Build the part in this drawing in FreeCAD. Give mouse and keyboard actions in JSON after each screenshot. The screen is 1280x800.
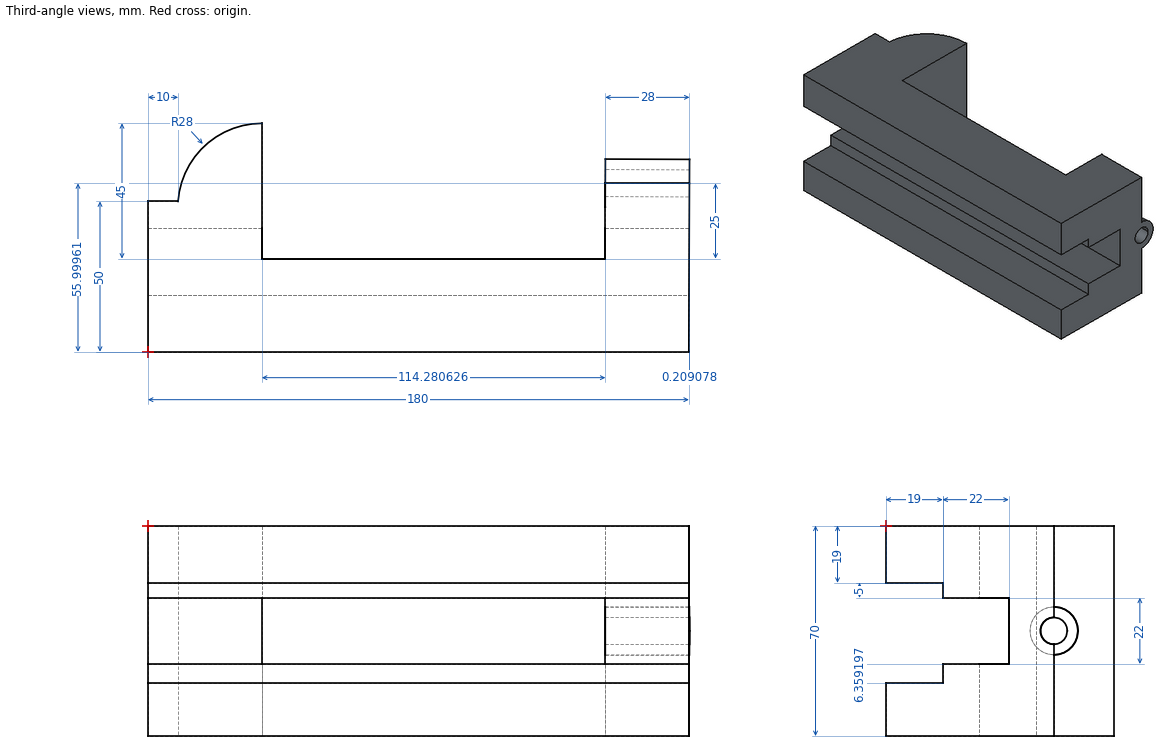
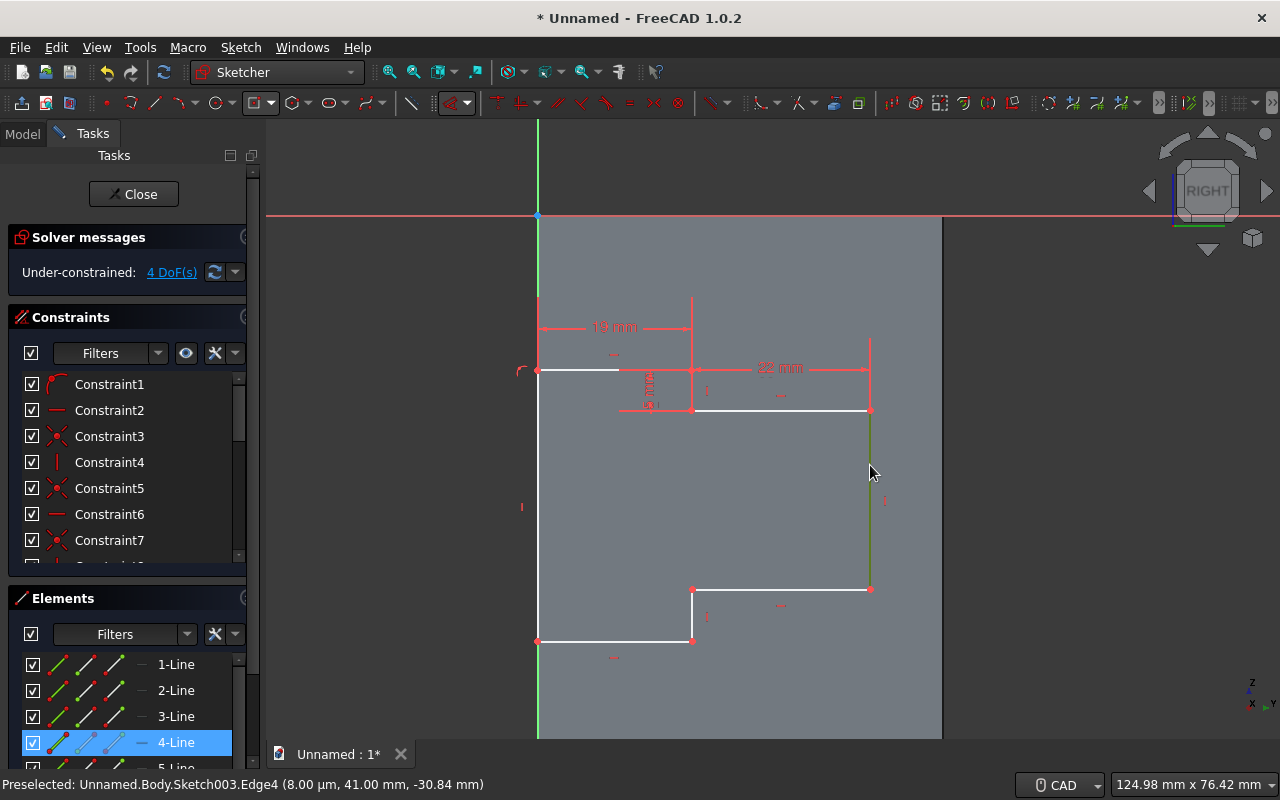
{"action": "key", "text": "i"}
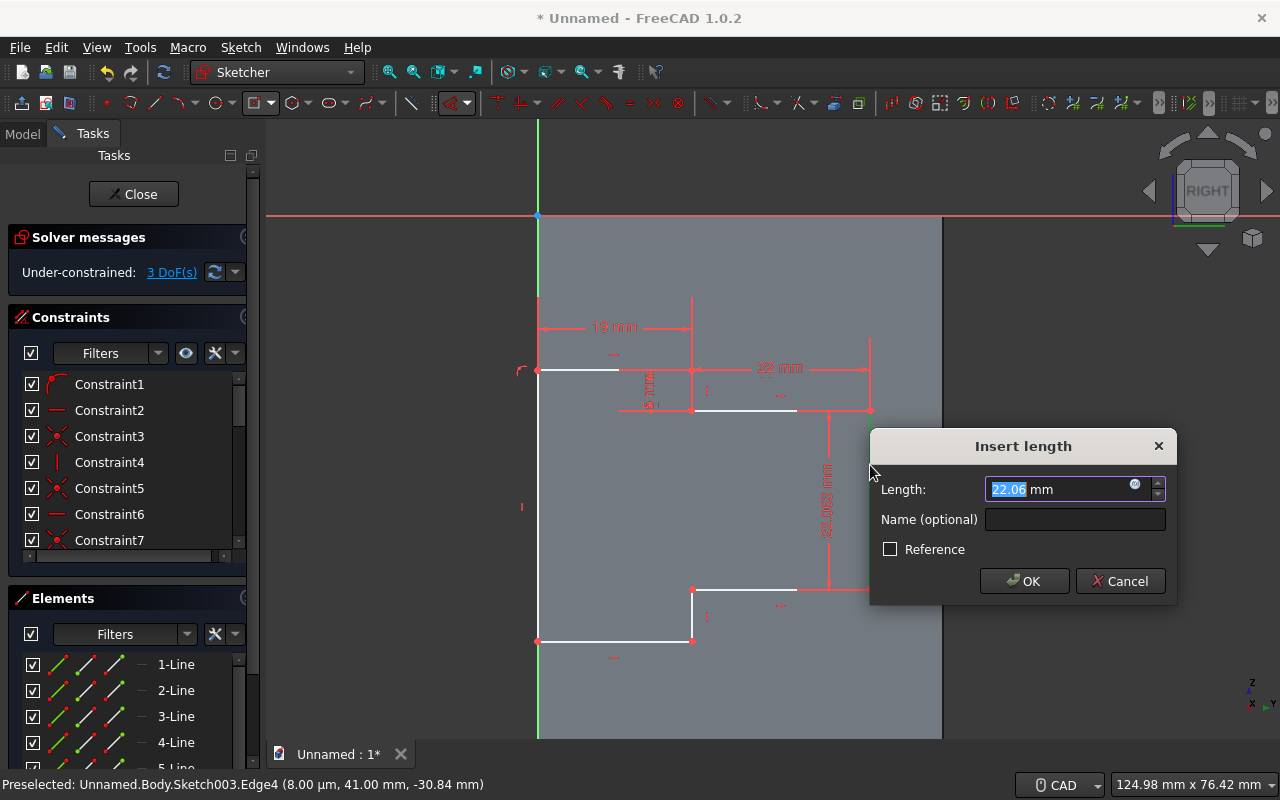
{"action": "type", "text": "22"}
{"action": "key", "text": "Return"}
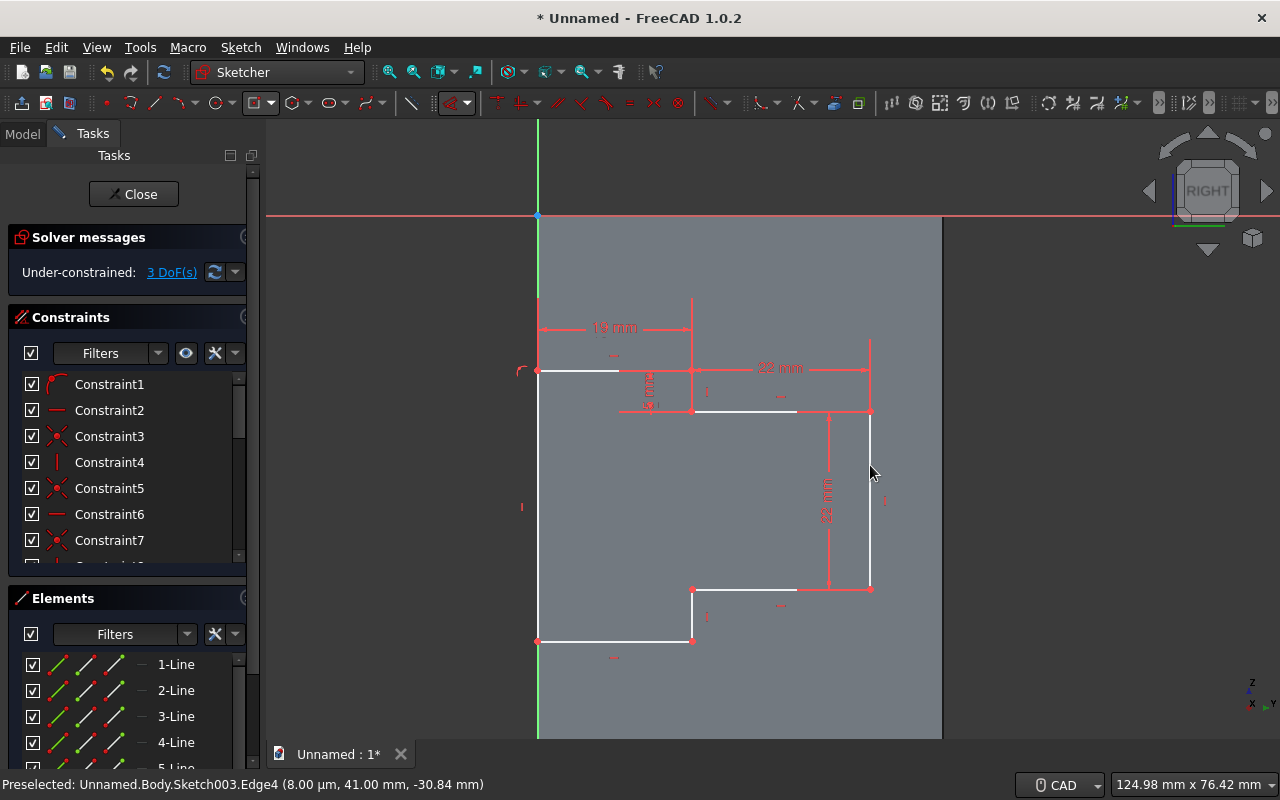
{"action": "left_click", "coordinate": [817, 590]}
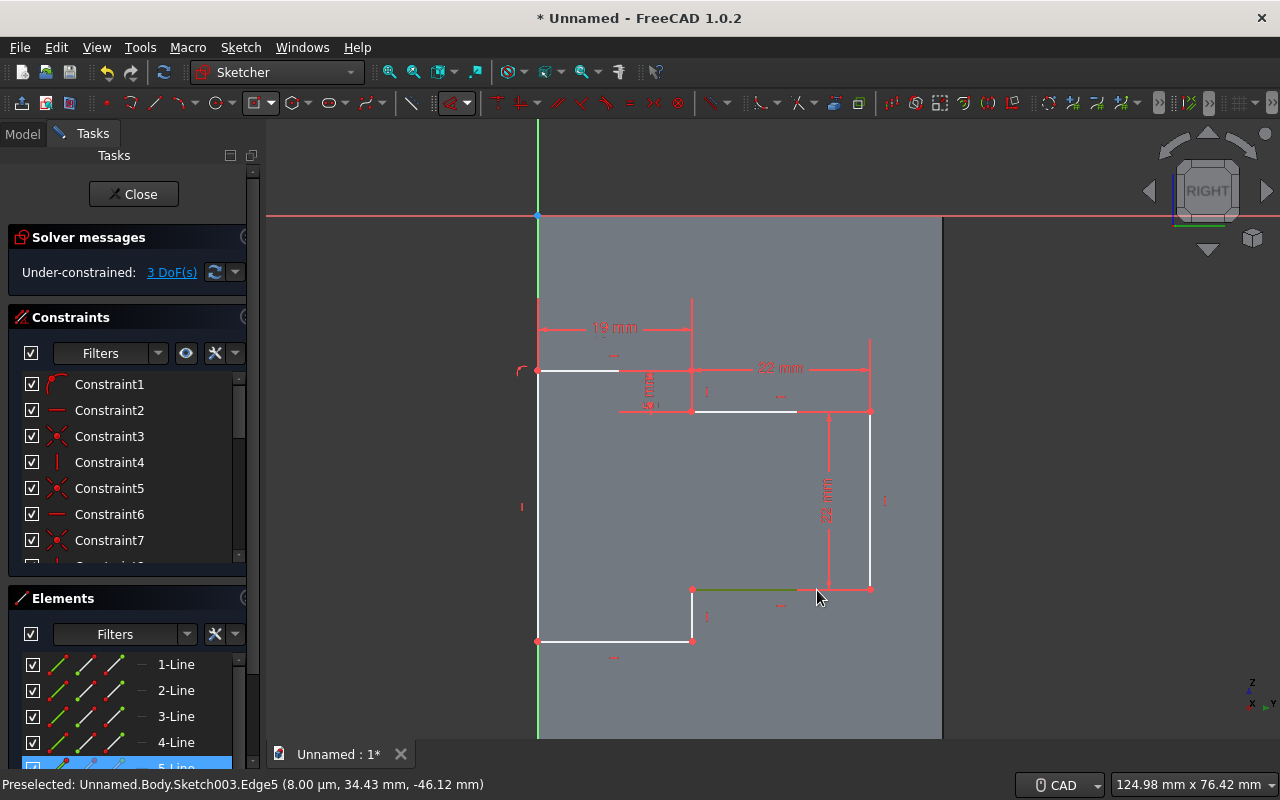
{"action": "left_click", "coordinate": [470, 104]}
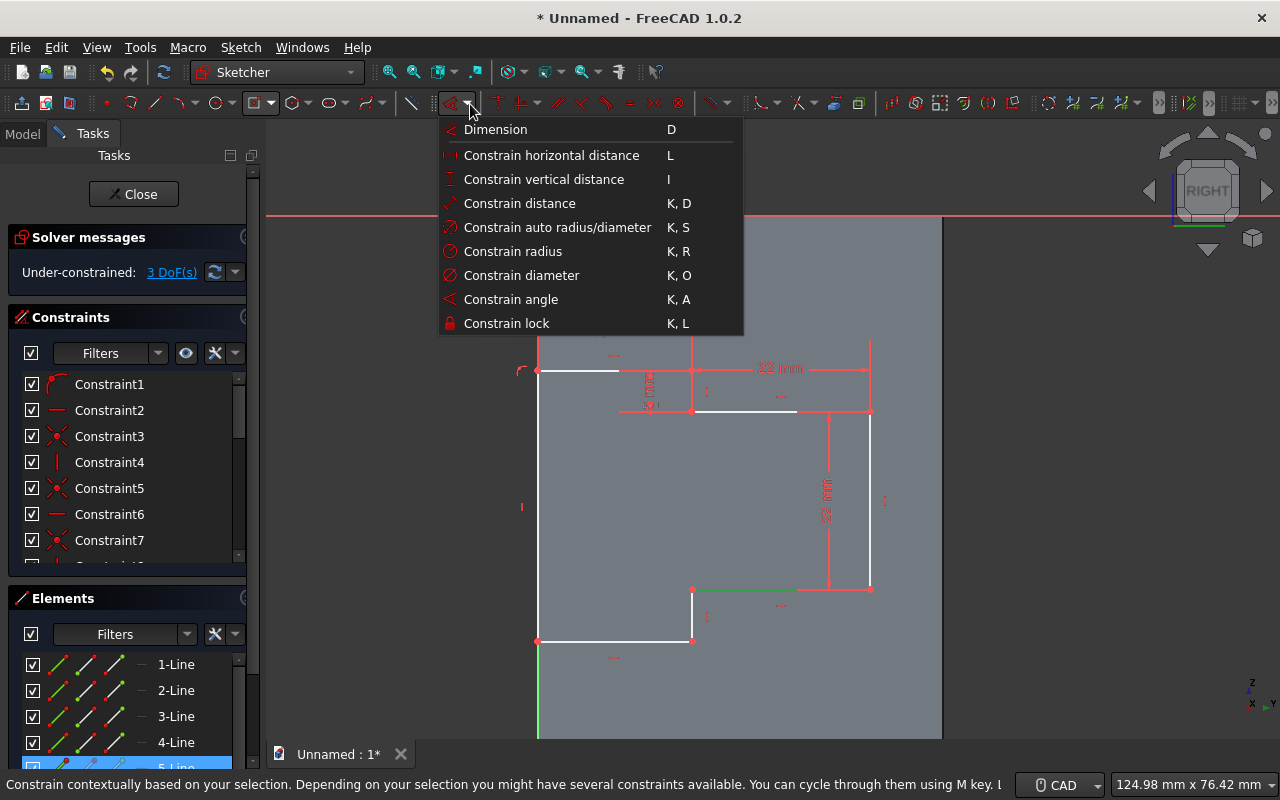
{"action": "left_click", "coordinate": [591, 155]}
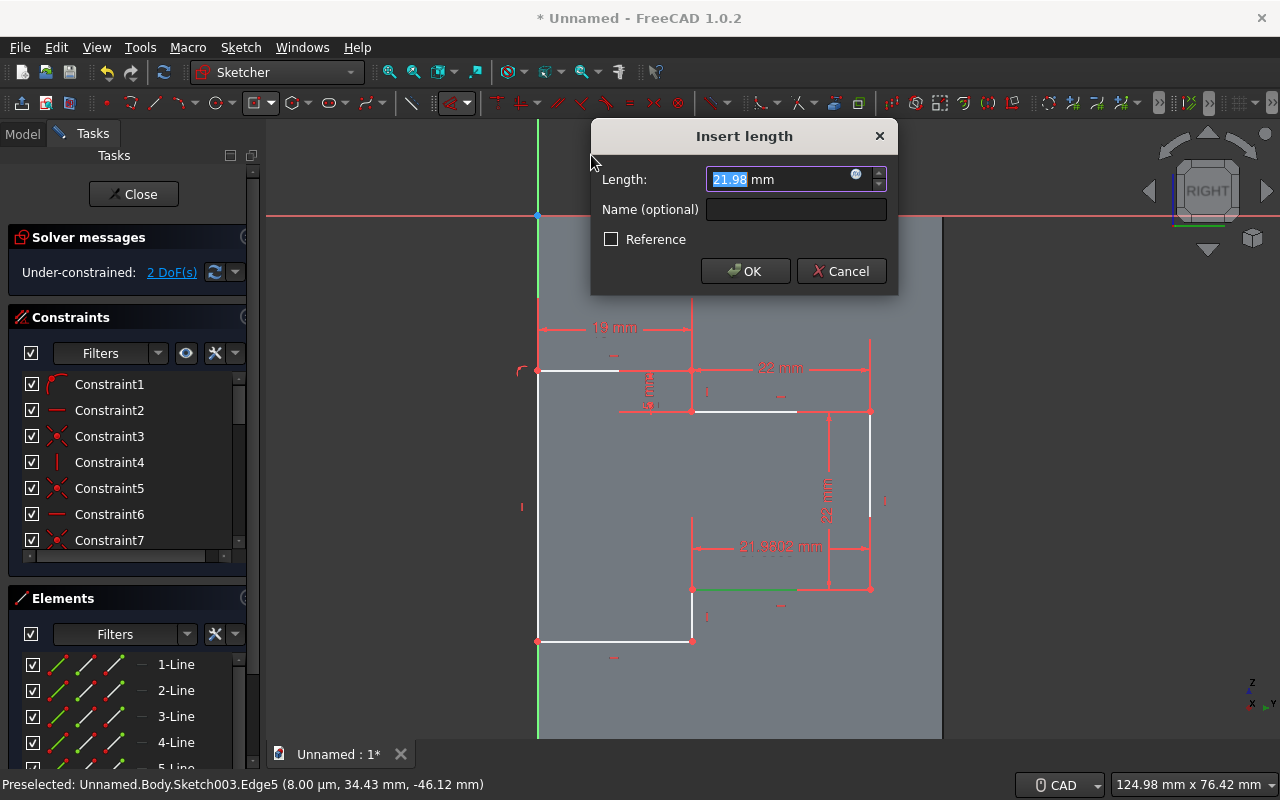
{"action": "type", "text": "22"}
{"action": "key", "text": "Return"}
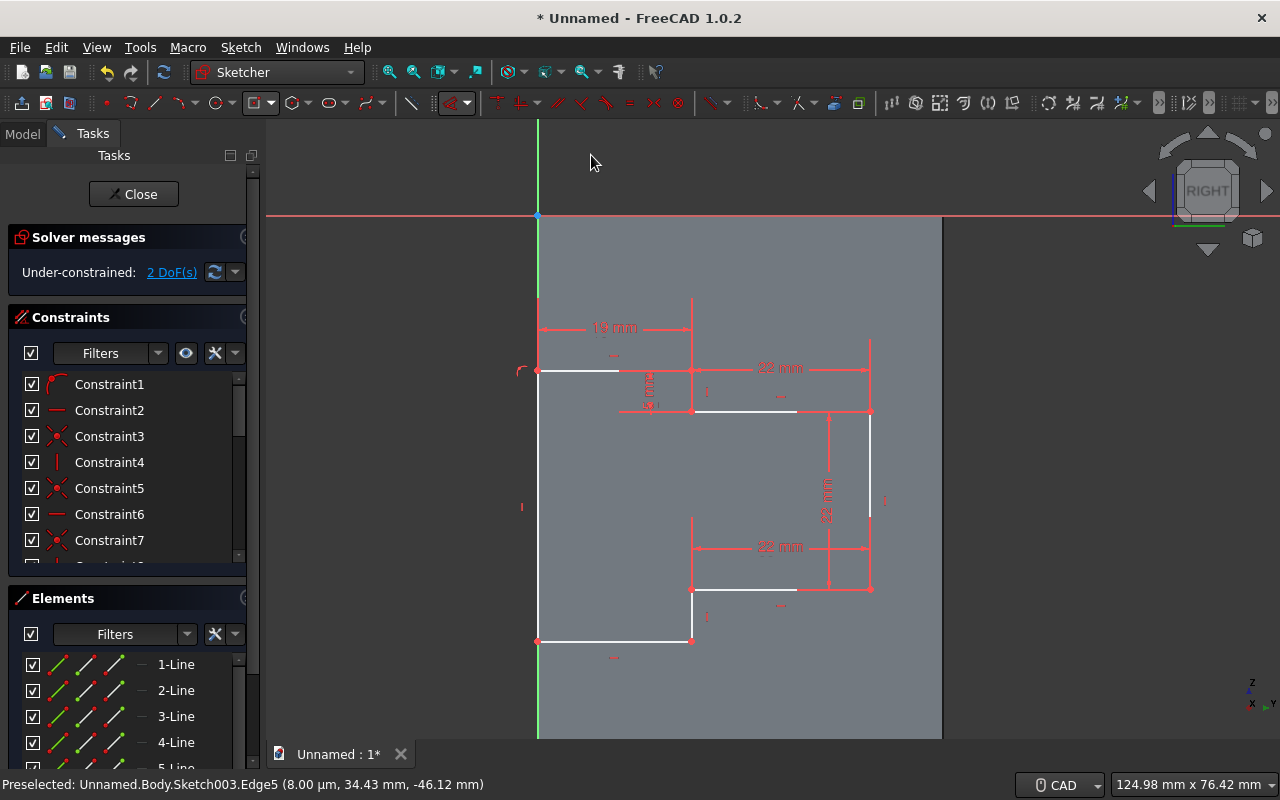
{"action": "left_click", "coordinate": [538, 371]}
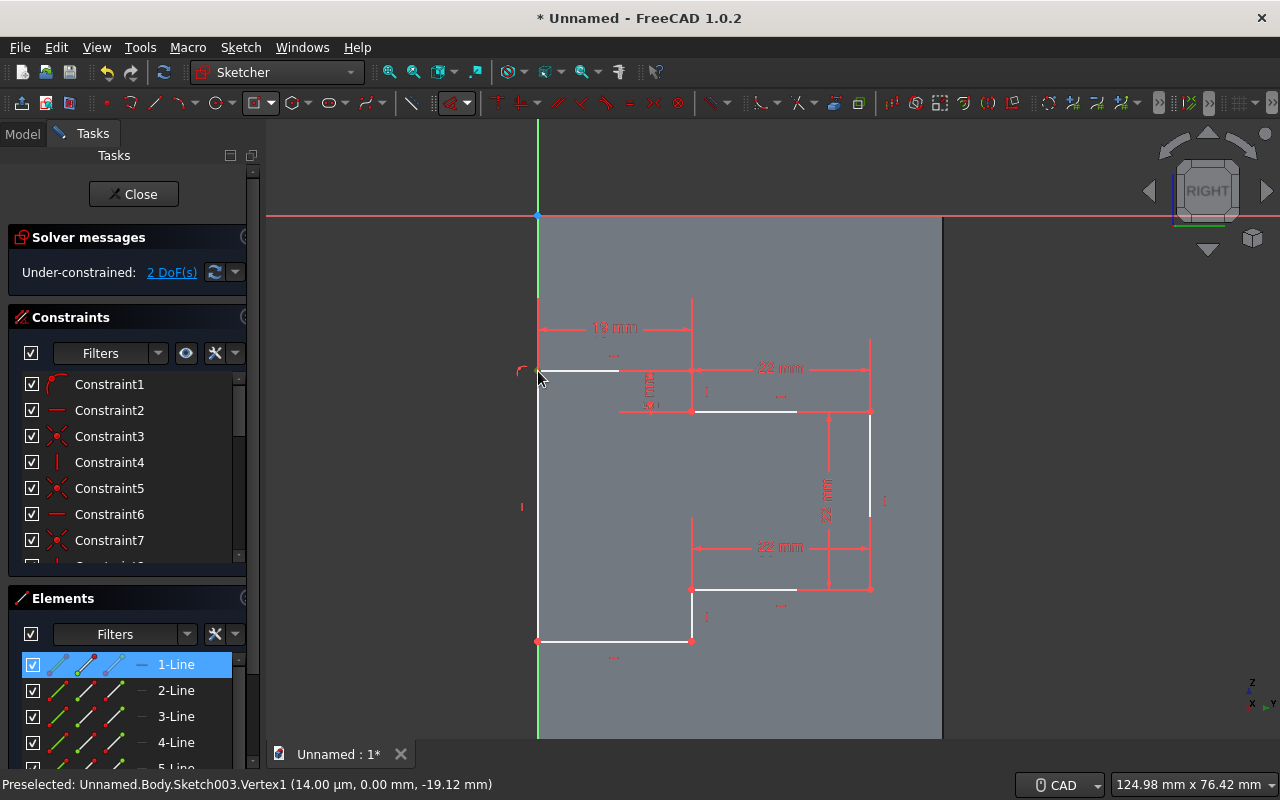
{"action": "left_click", "coordinate": [470, 104]}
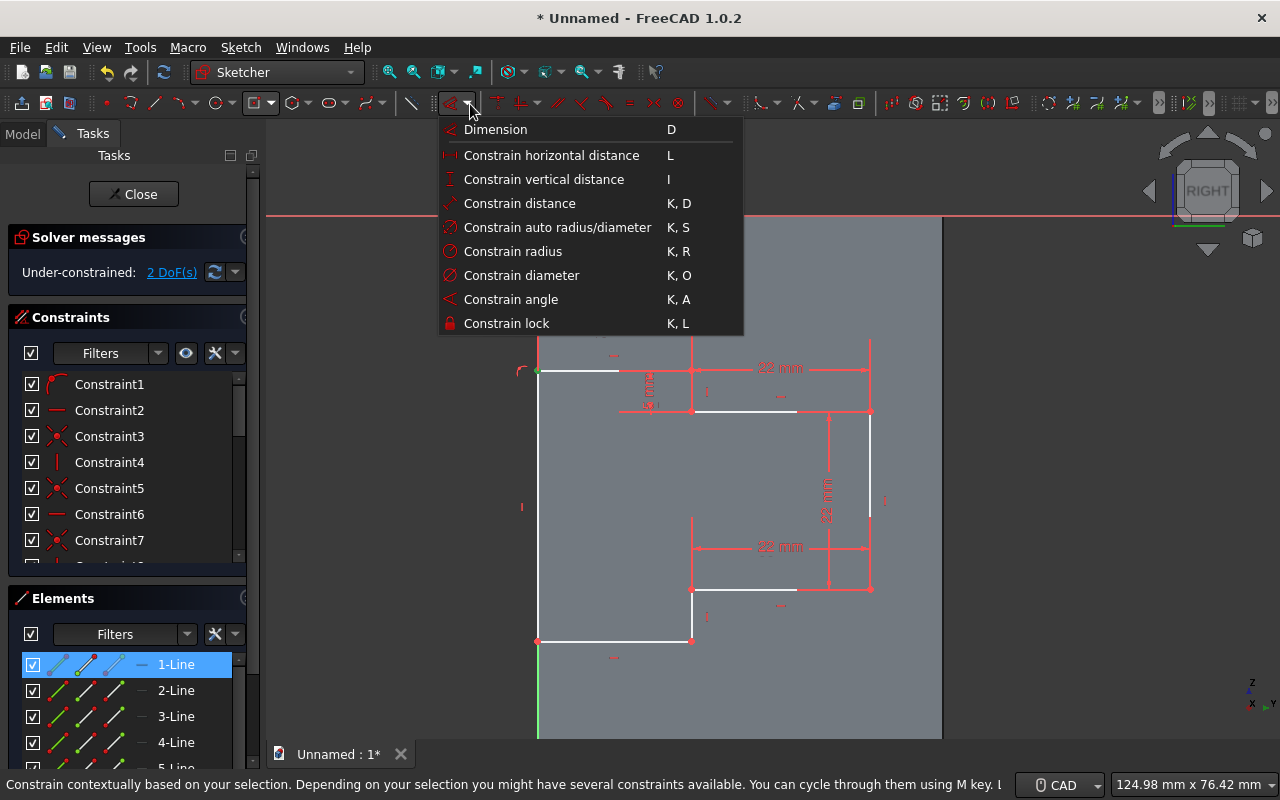
{"action": "left_click", "coordinate": [591, 179]}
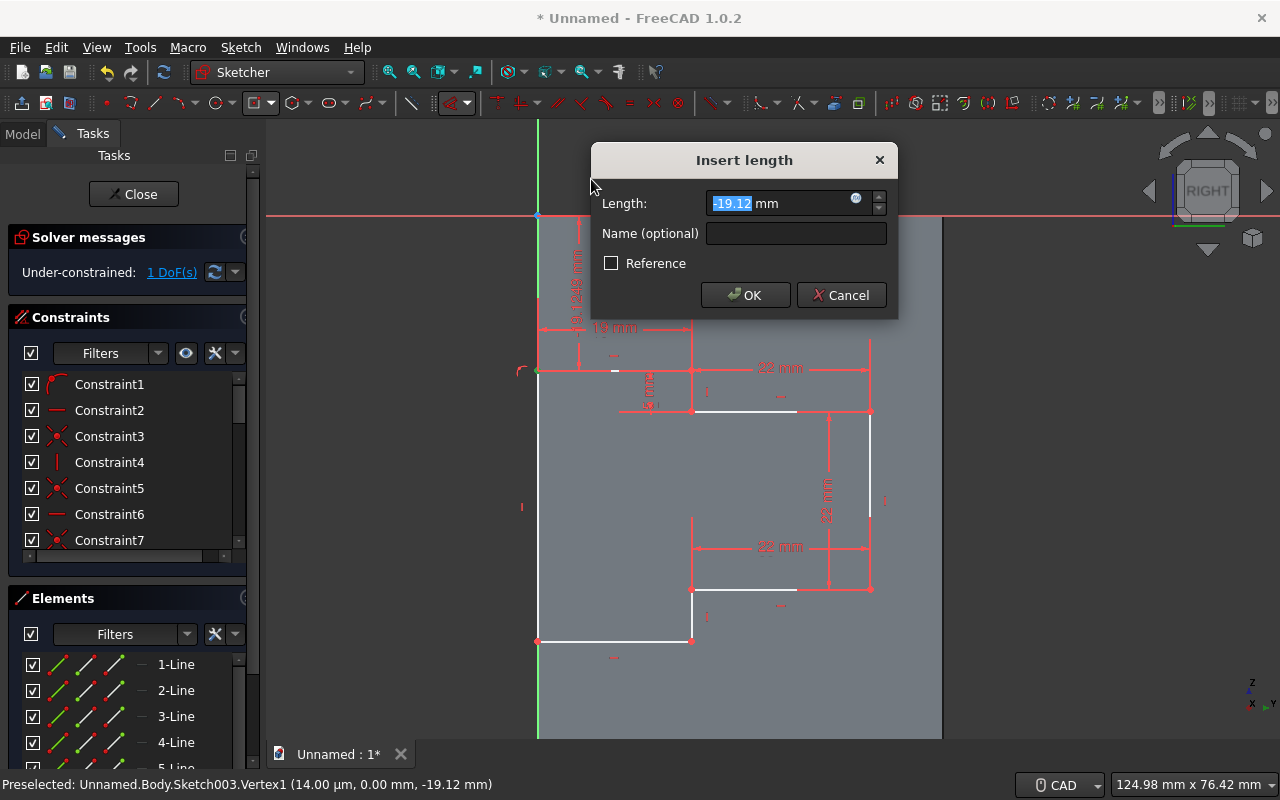
{"action": "type", "text": "-19"}
{"action": "key", "text": "Return"}